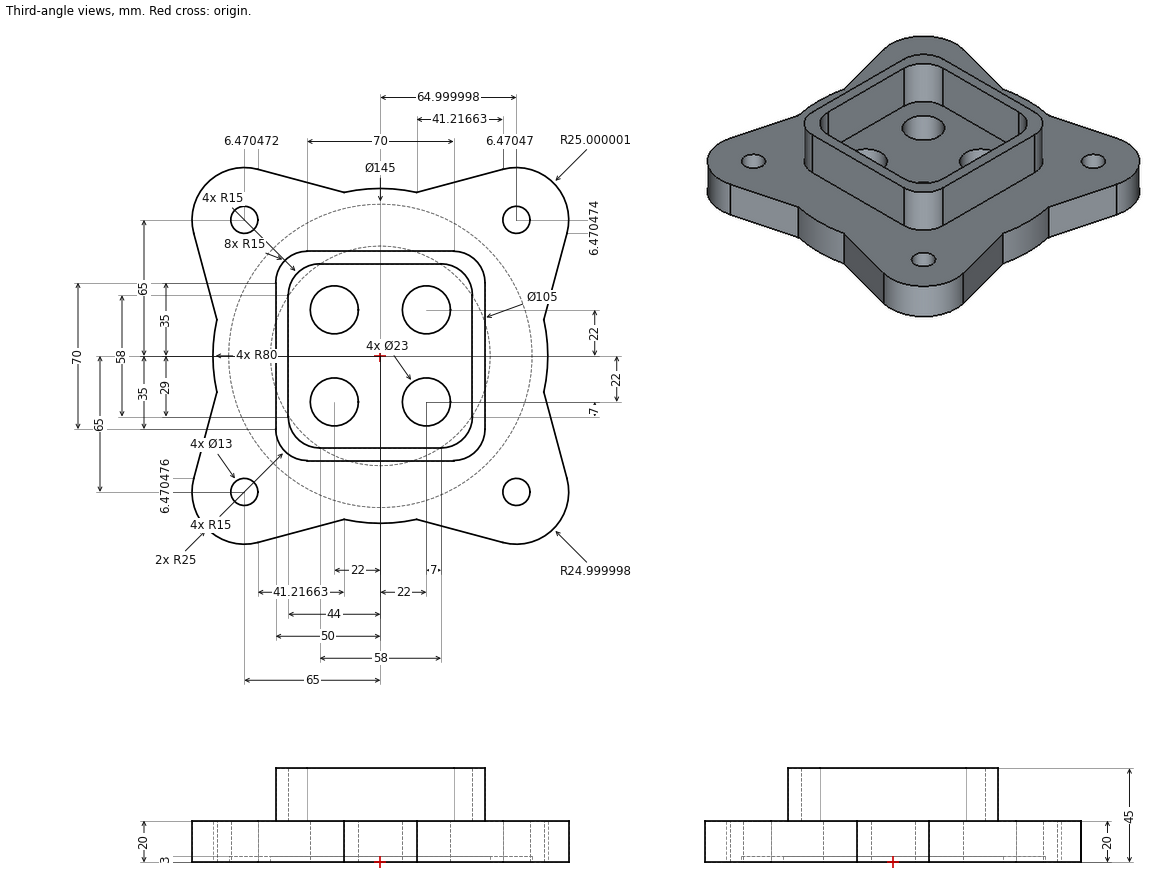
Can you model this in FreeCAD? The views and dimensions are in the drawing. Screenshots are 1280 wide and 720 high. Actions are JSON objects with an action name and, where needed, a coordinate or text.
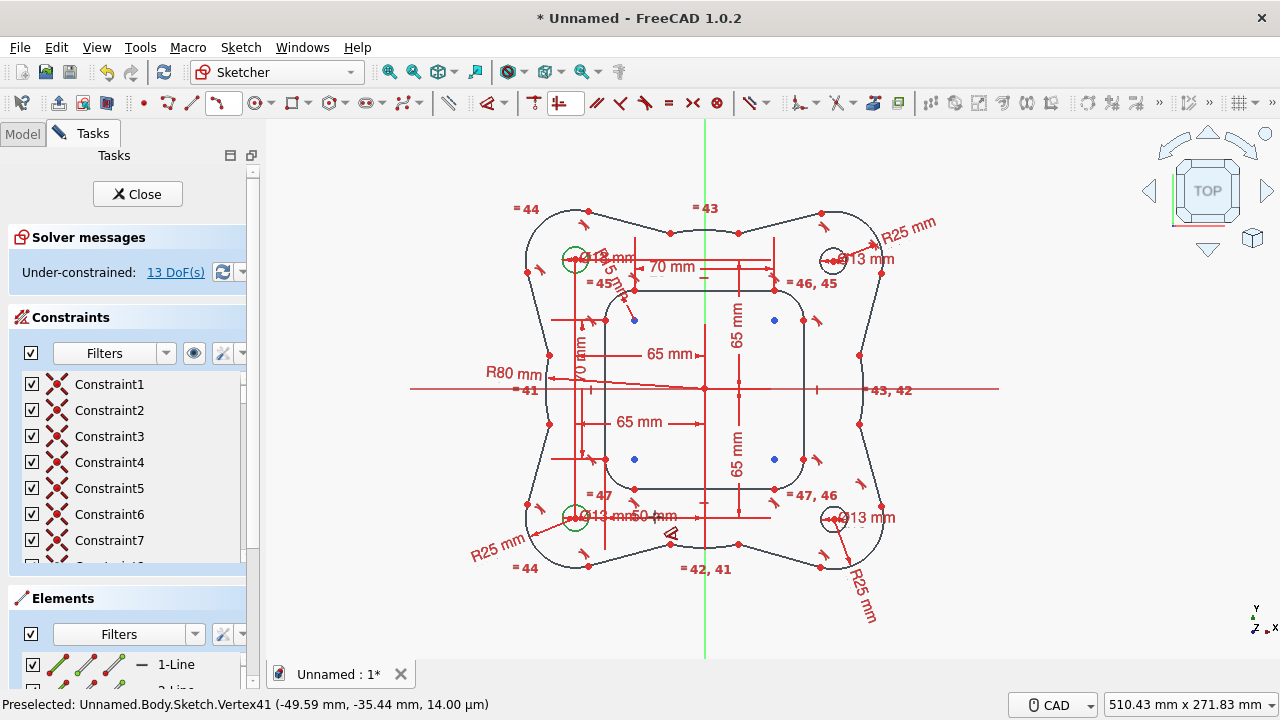
{"action": "left_click", "coordinate": [605, 459]}
{"action": "left_click", "coordinate": [571, 449]}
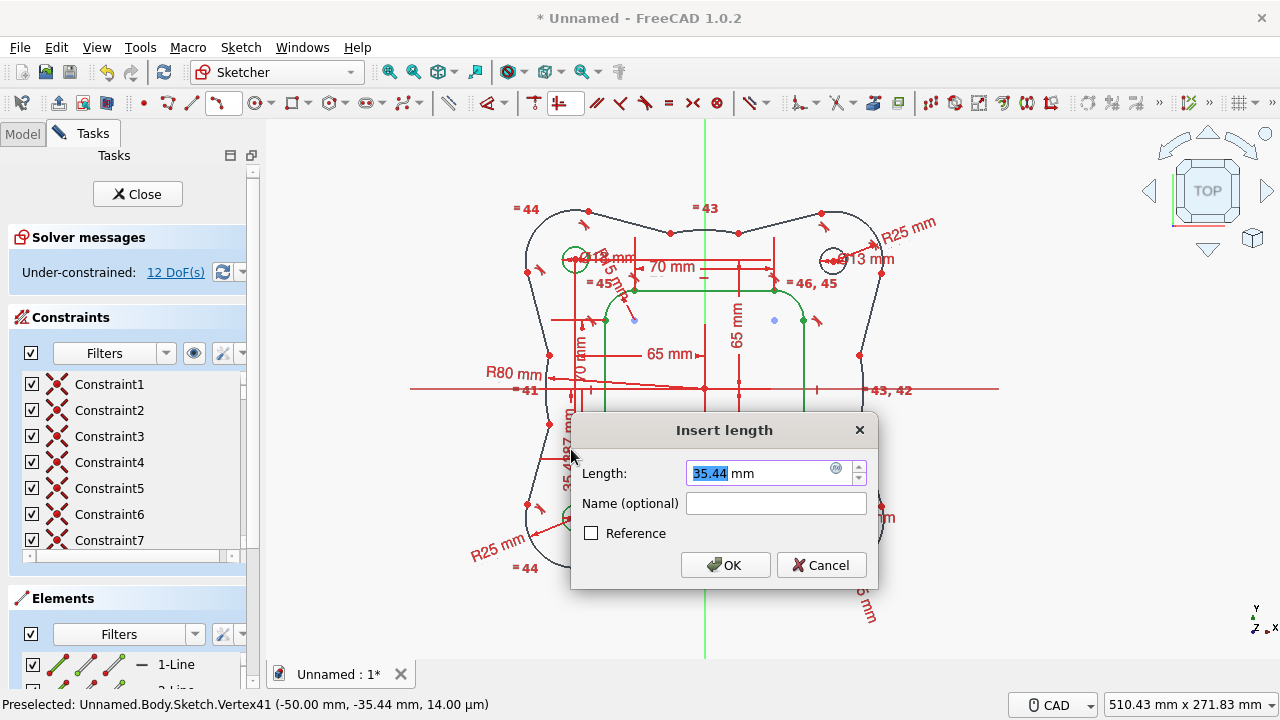
{"action": "type", "text": "35"}
{"action": "key", "text": "Return"}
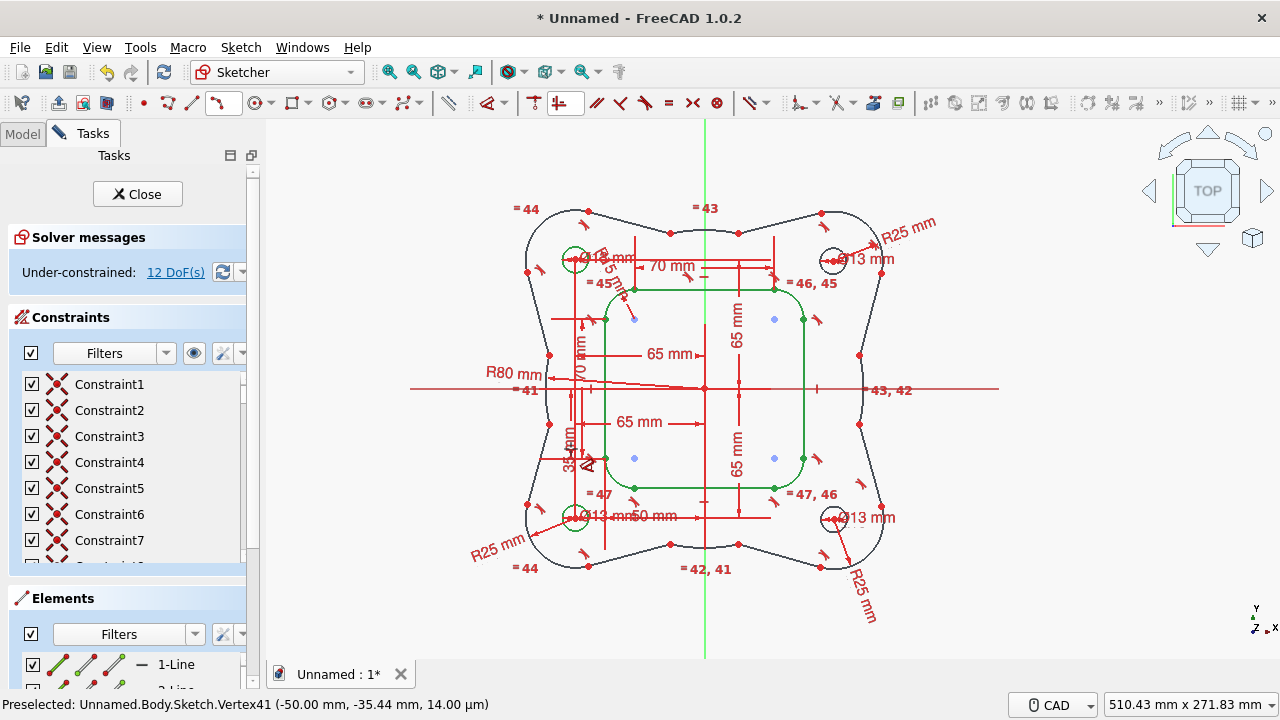
{"action": "scroll", "coordinate": [821, 213], "scroll_direction": "up", "scroll_amount": 6}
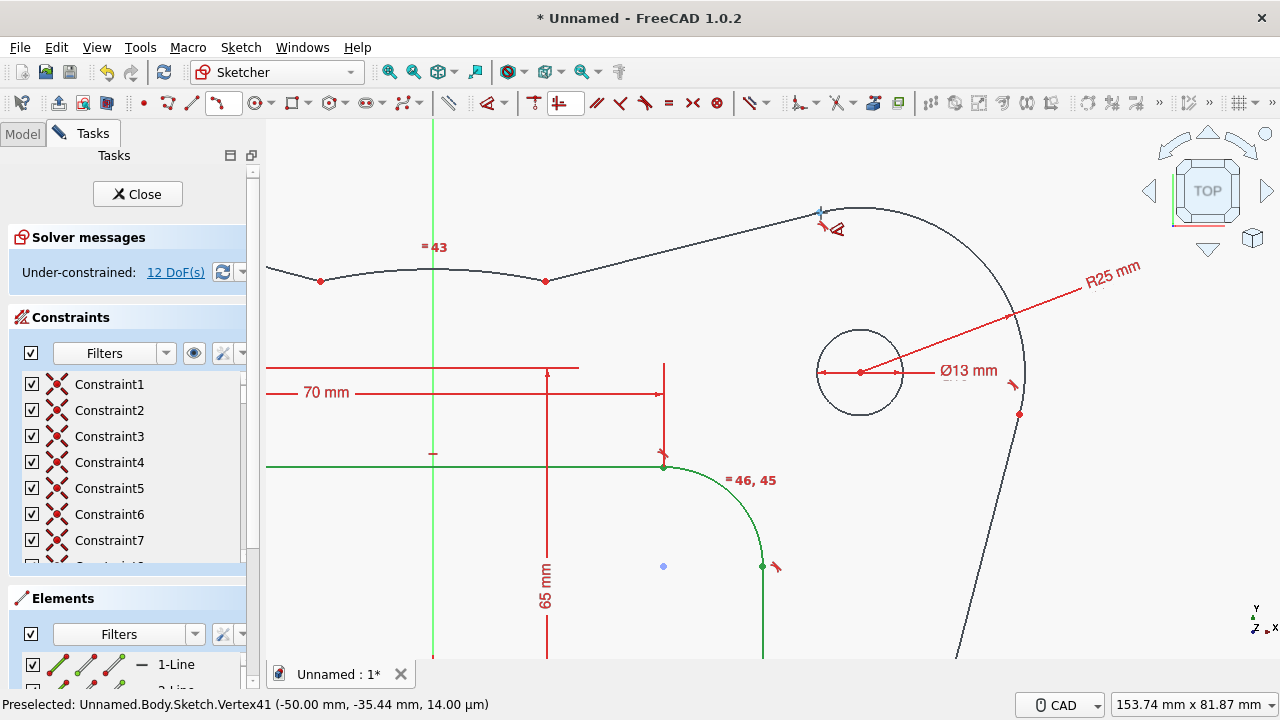
{"action": "left_click", "coordinate": [820, 213]}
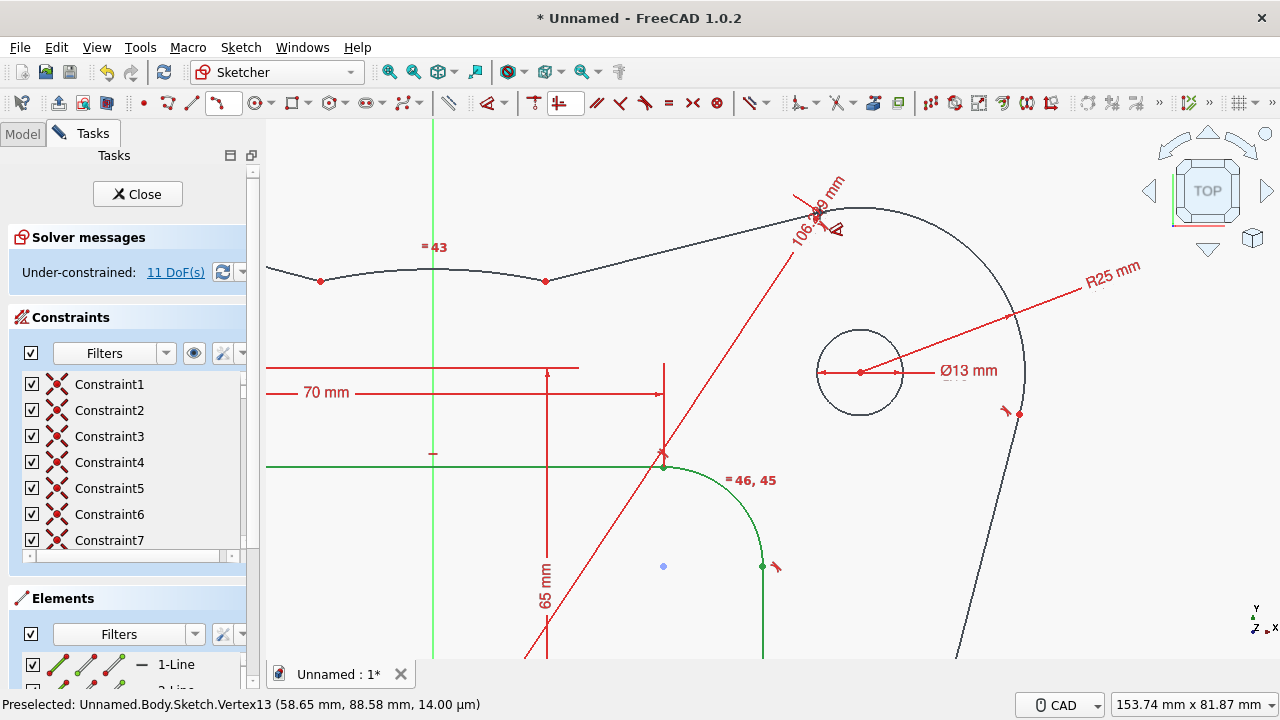
{"action": "left_click", "coordinate": [860, 373]}
{"action": "left_click", "coordinate": [840, 179]}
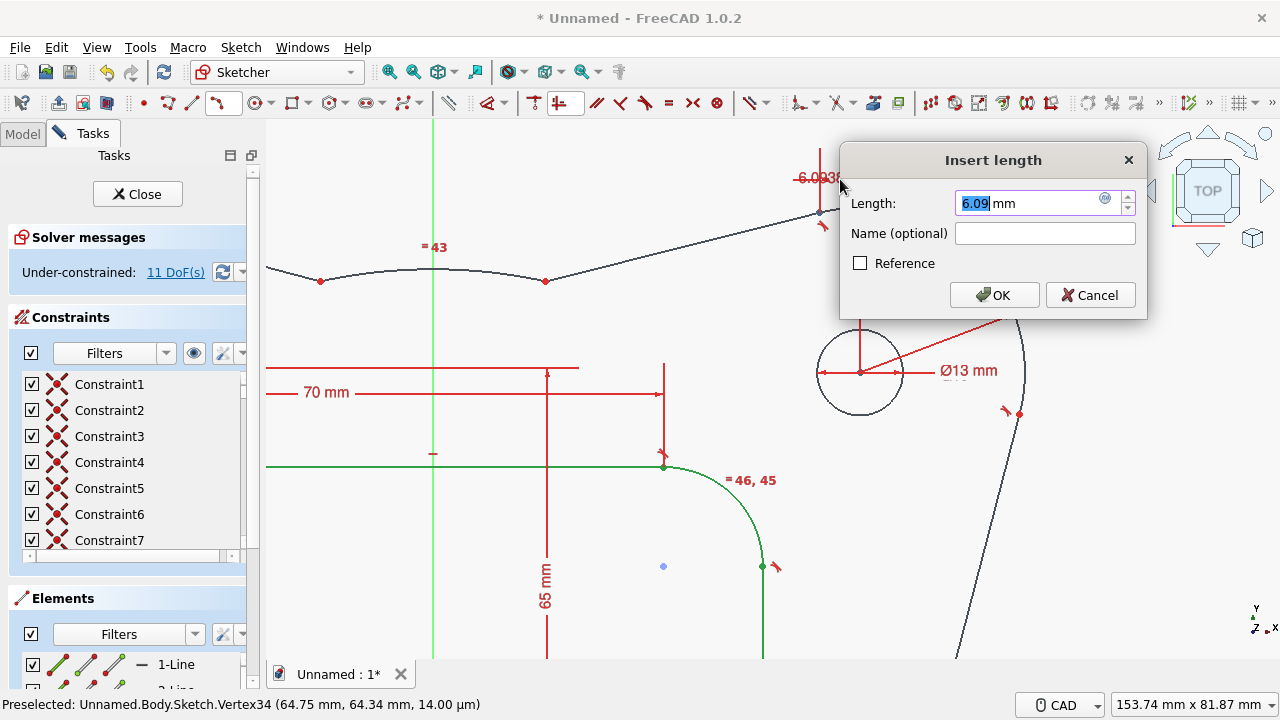
{"action": "type", "text": "6.47047"}
{"action": "key", "text": "Return"}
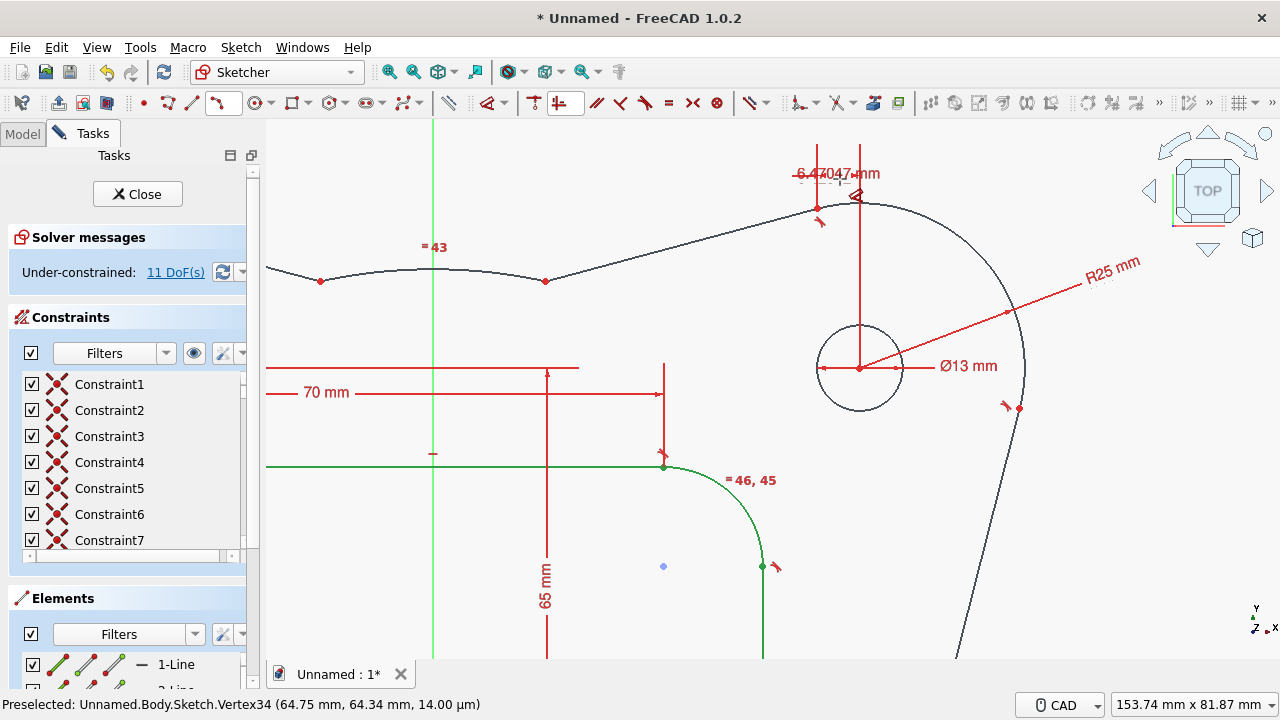
{"action": "scroll", "coordinate": [822, 213], "scroll_direction": "down", "scroll_amount": 6}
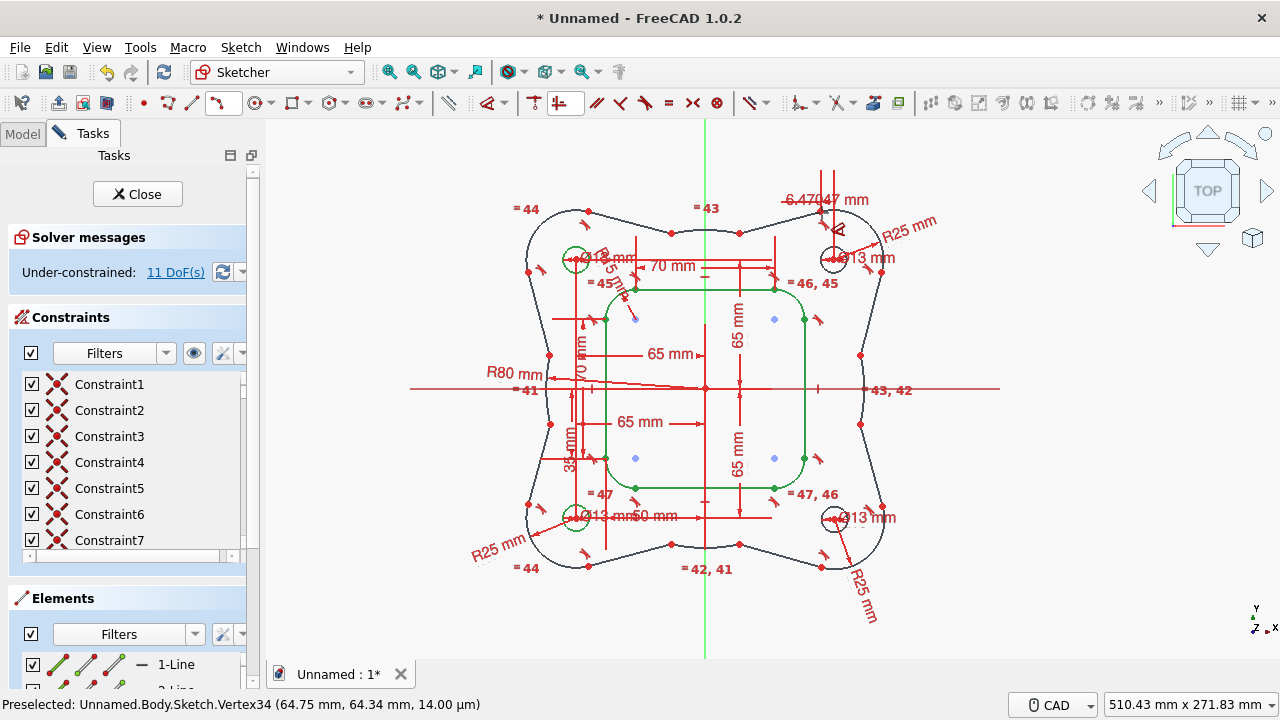
{"action": "left_click", "coordinate": [614, 560]}
{"action": "left_click", "coordinate": [630, 600]}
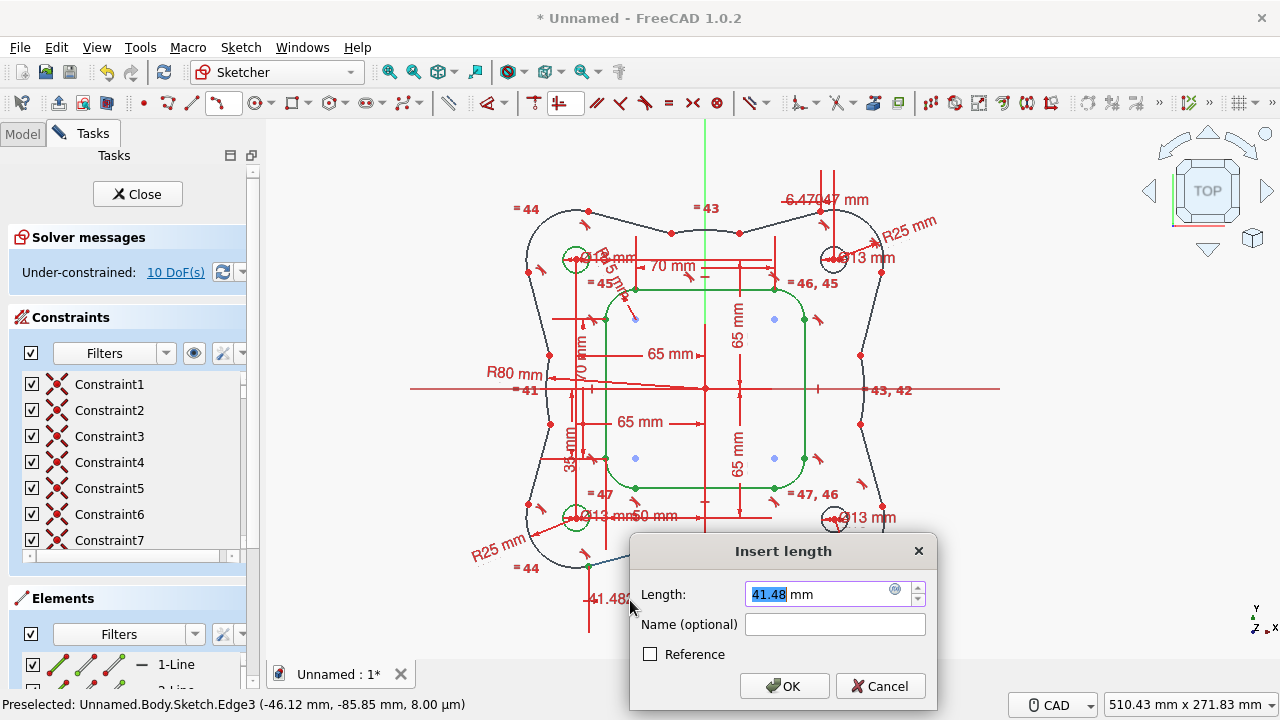
{"action": "type", "text": "41.21663"}
{"action": "key", "text": "Return"}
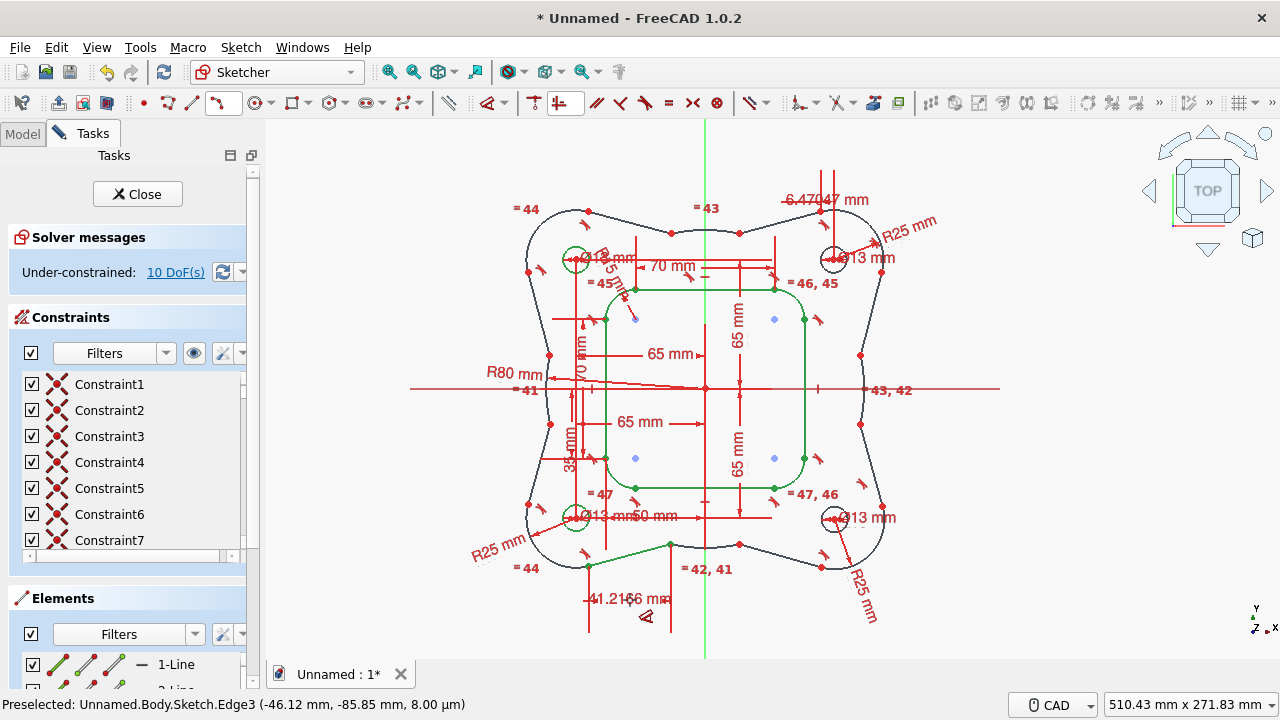
{"action": "left_click", "coordinate": [796, 218]}
{"action": "left_click", "coordinate": [780, 178]}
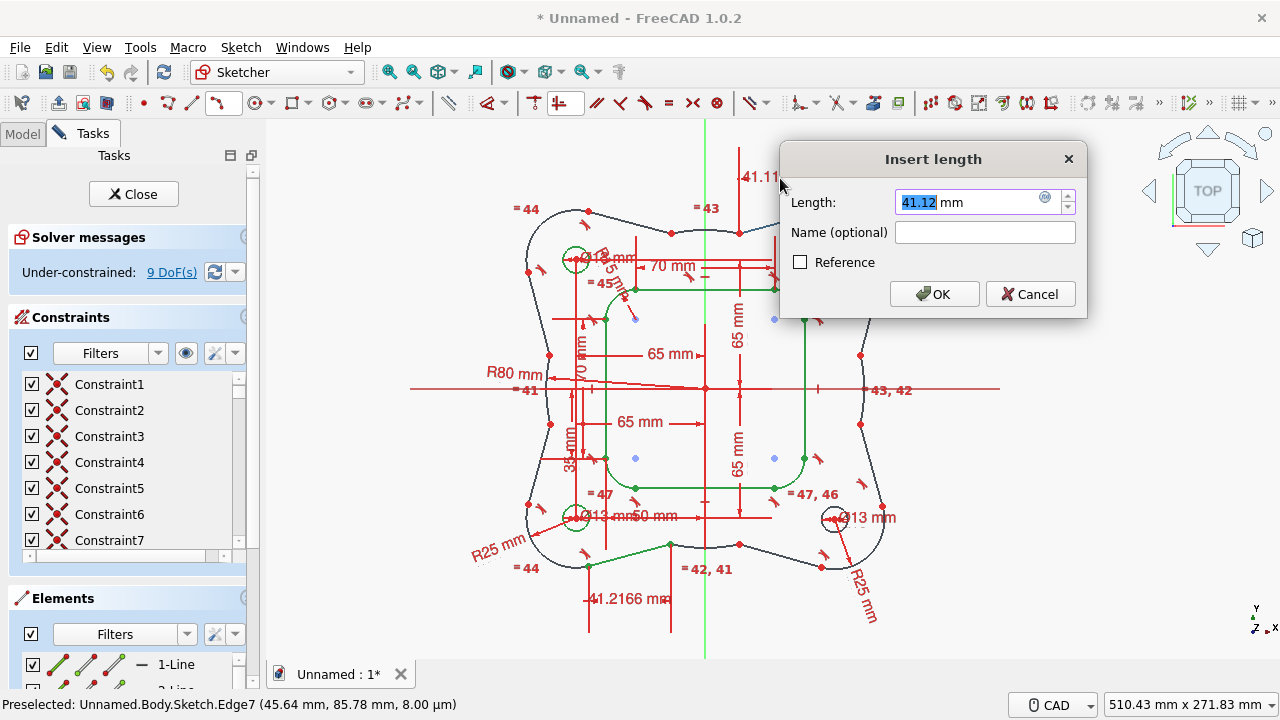
{"action": "type", "text": "41.21663"}
{"action": "key", "text": "Return"}